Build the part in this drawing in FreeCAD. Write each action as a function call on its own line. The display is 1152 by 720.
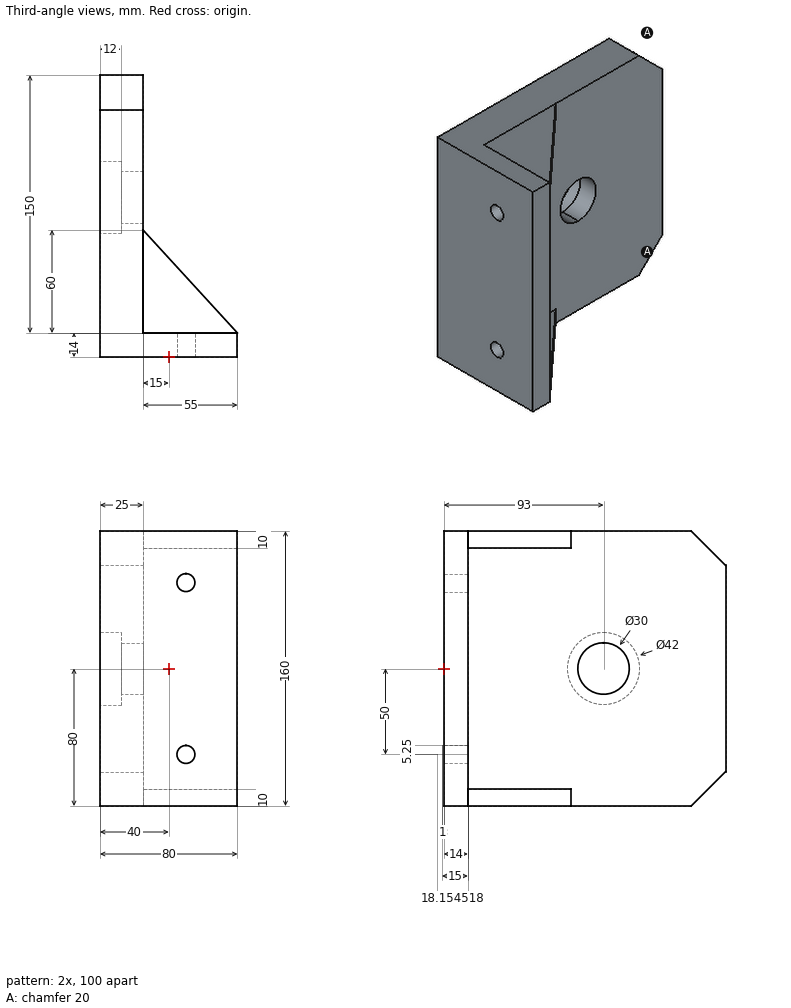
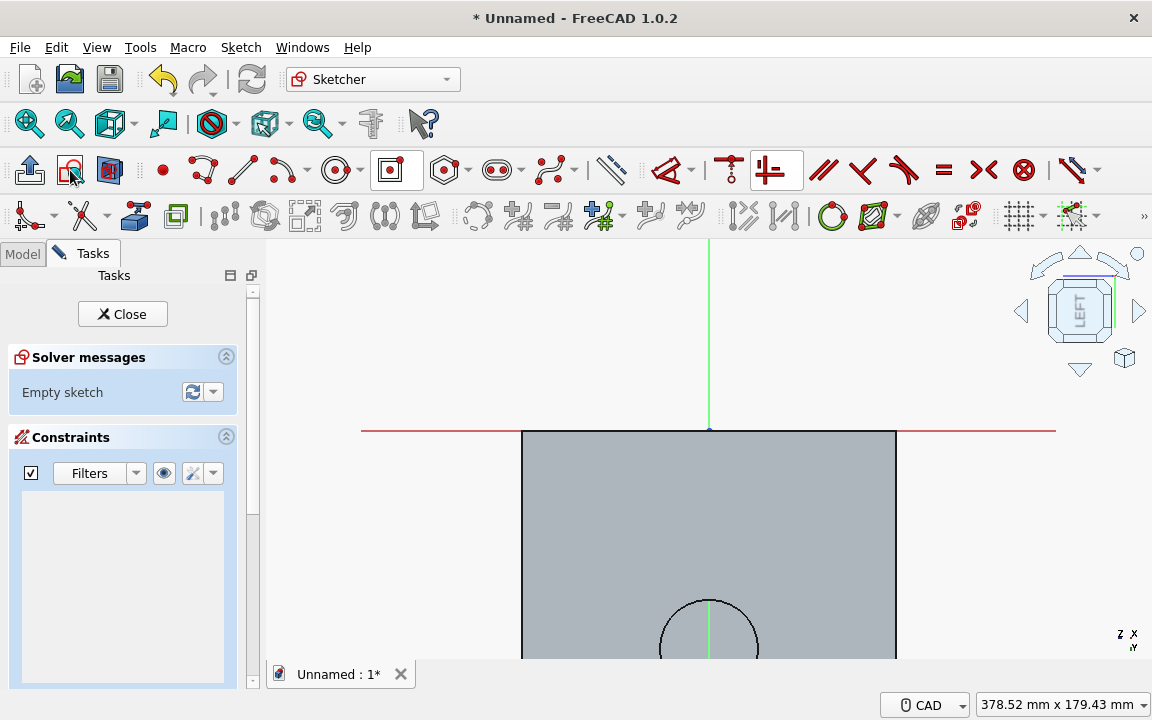
scroll(640, 449, down, 5)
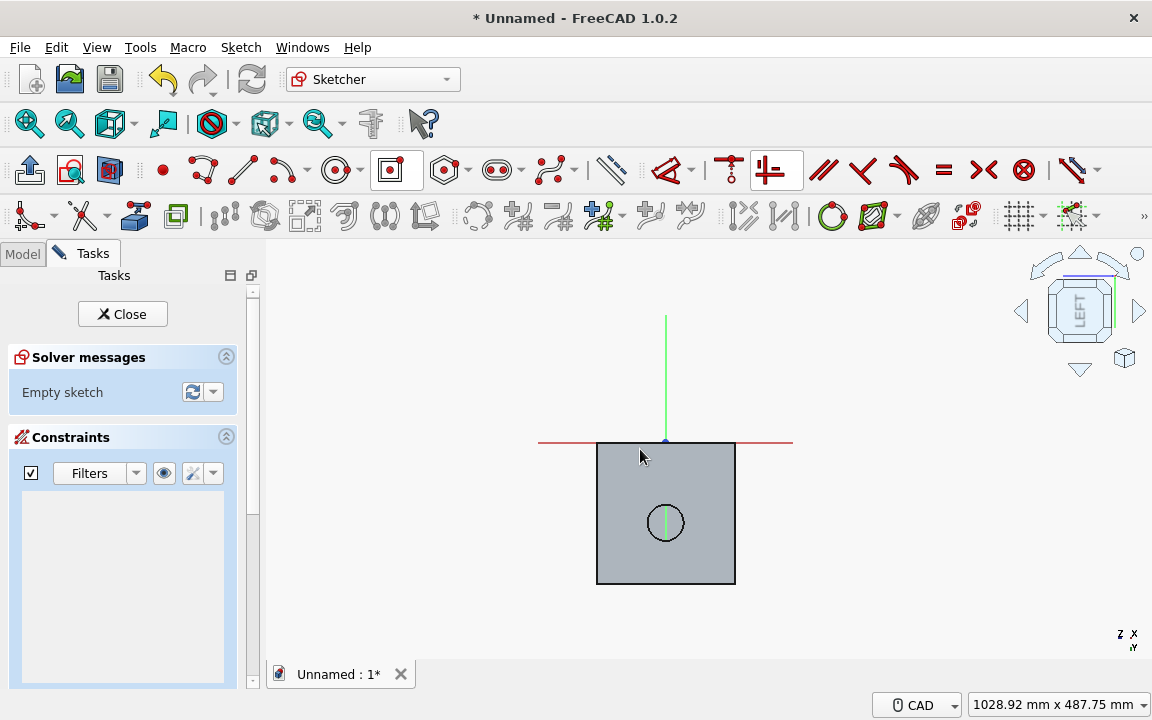
scroll(669, 532, up, 11)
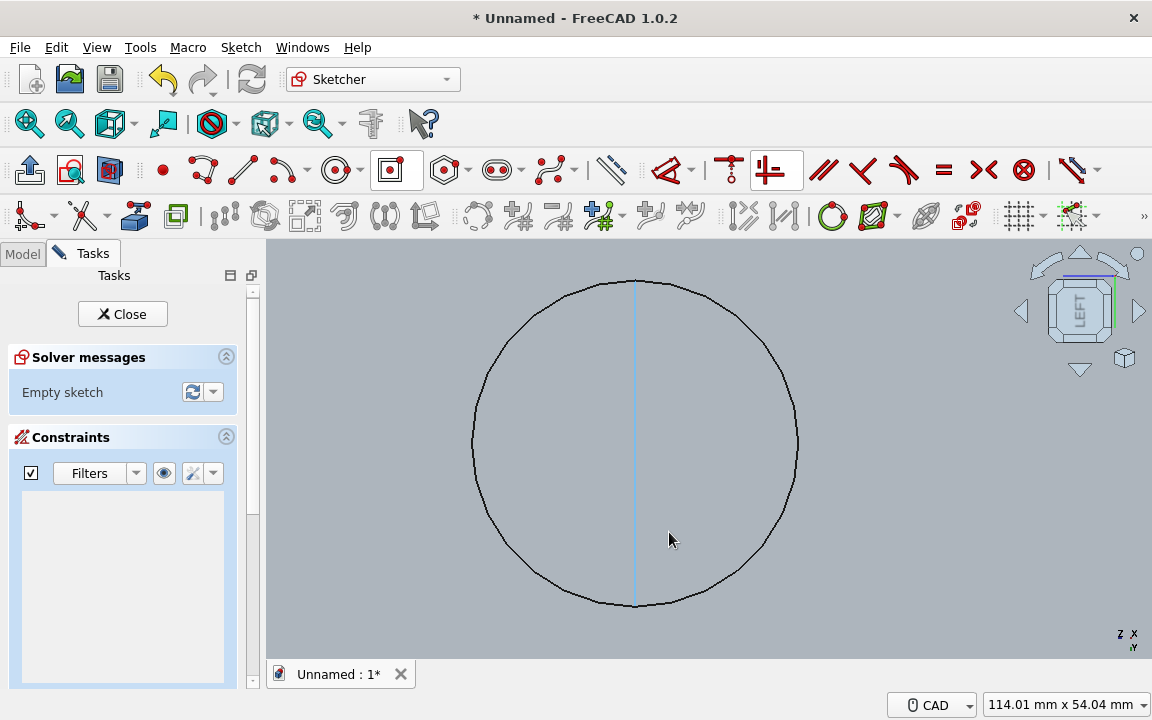
click(336, 170)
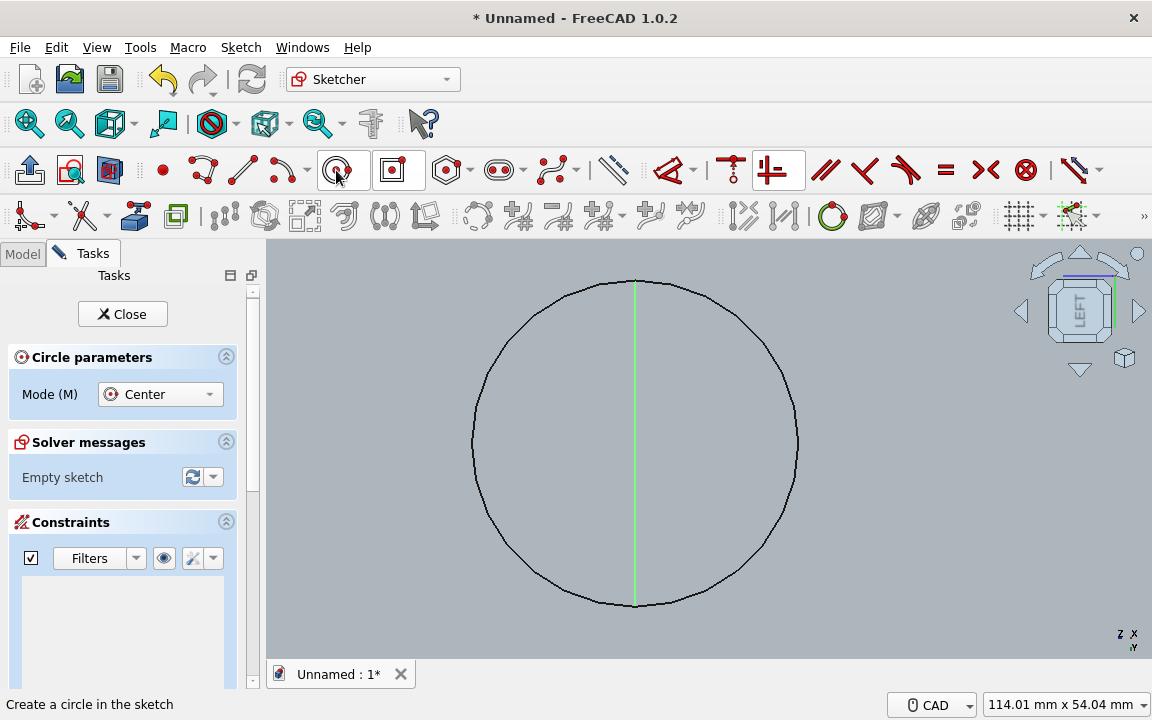
click(635, 444)
move(718, 361)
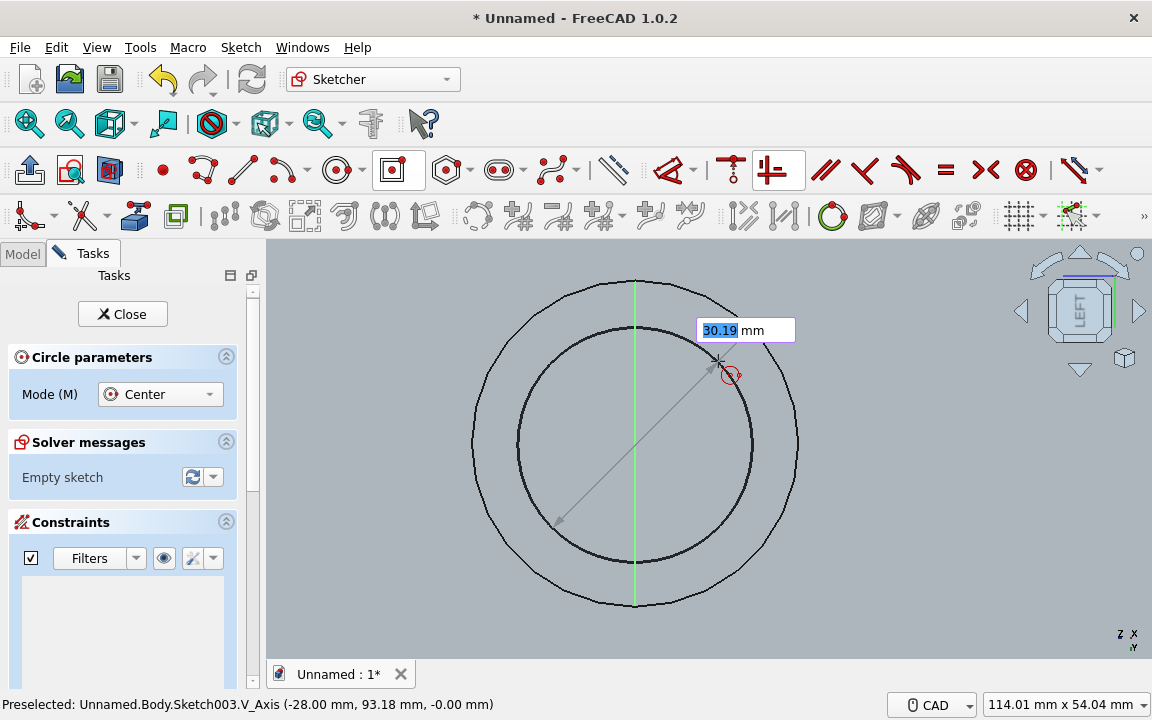
text(30)
key(Return)
key(Escape)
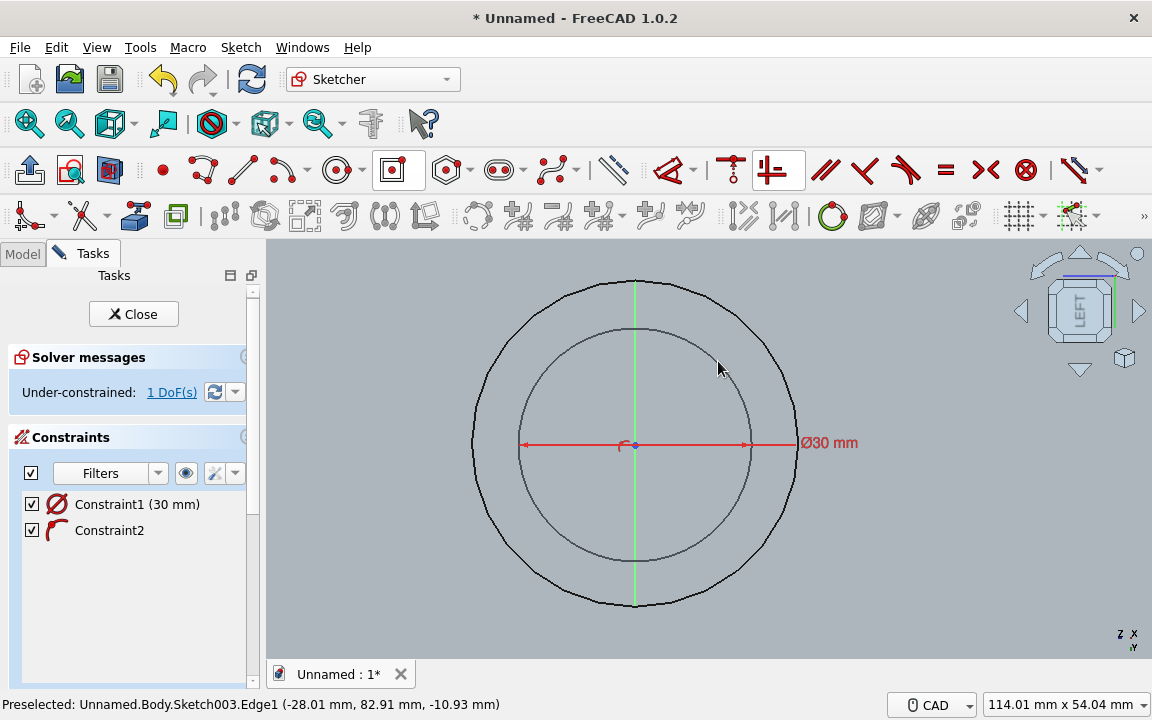
click(668, 170)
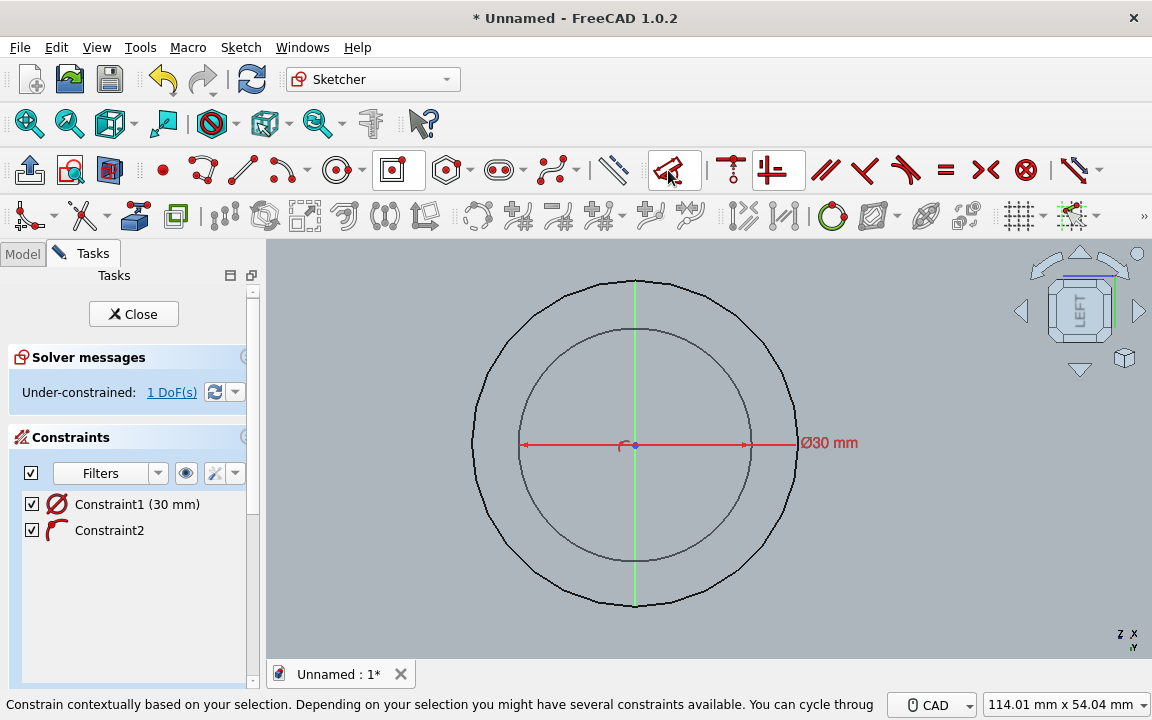
click(635, 445)
click(669, 356)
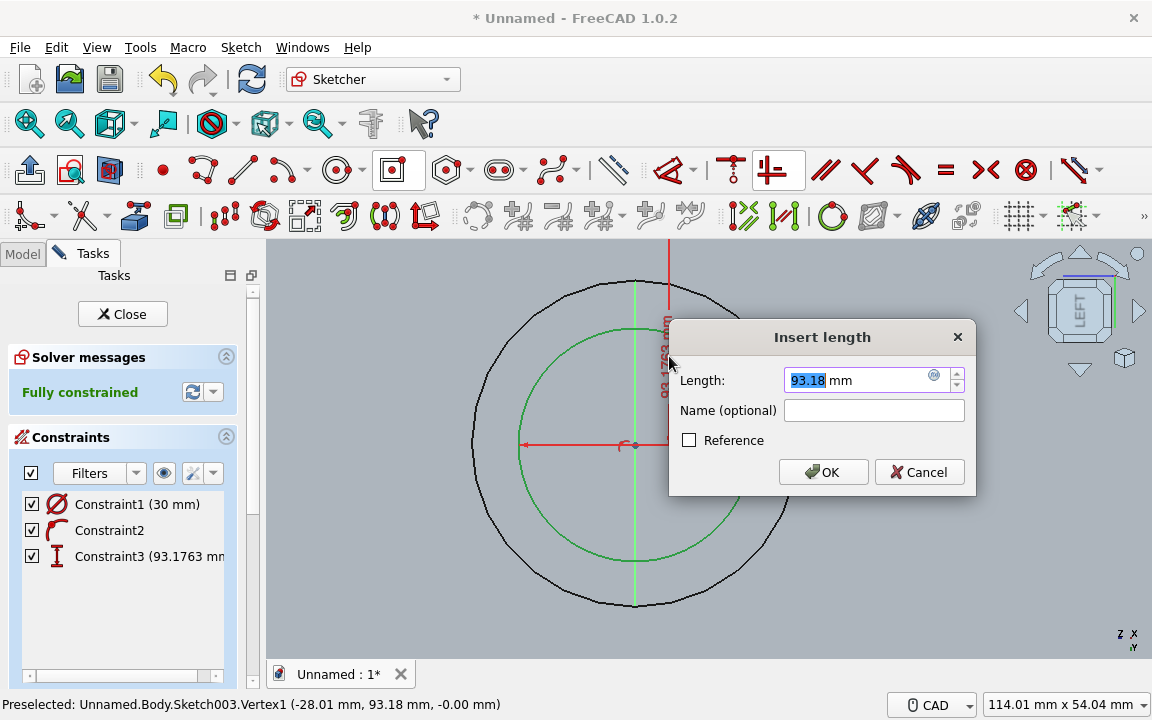
text(93)
key(Return)
key(Escape)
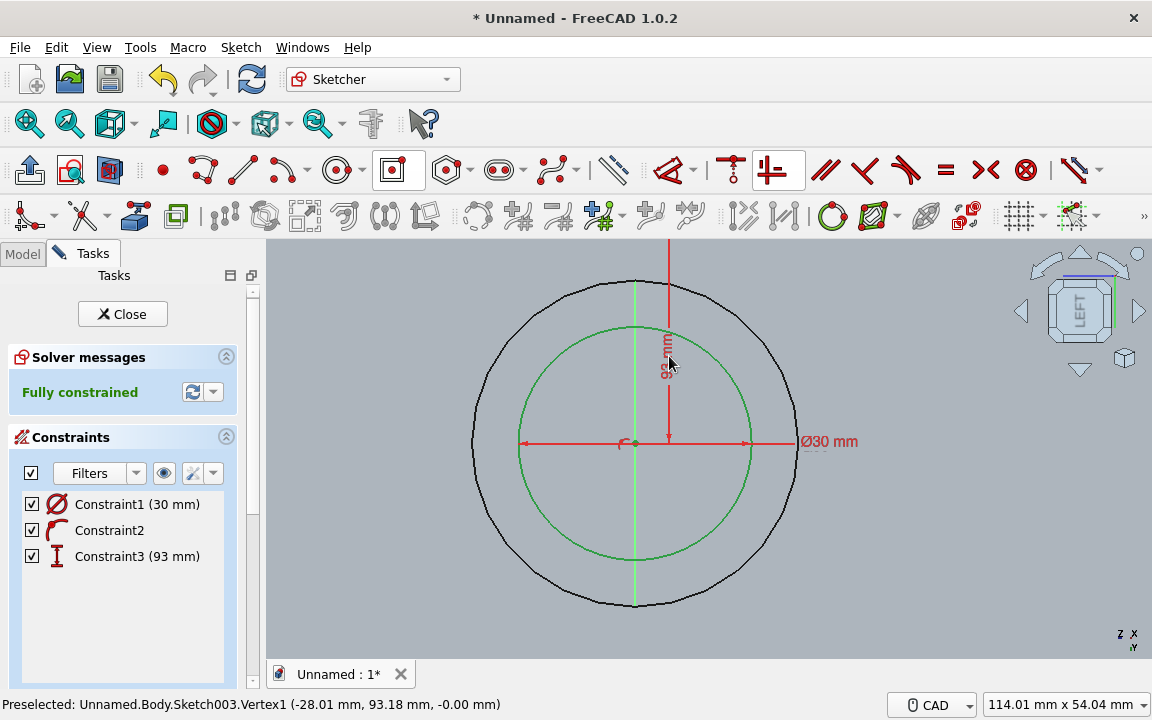
click(123, 314)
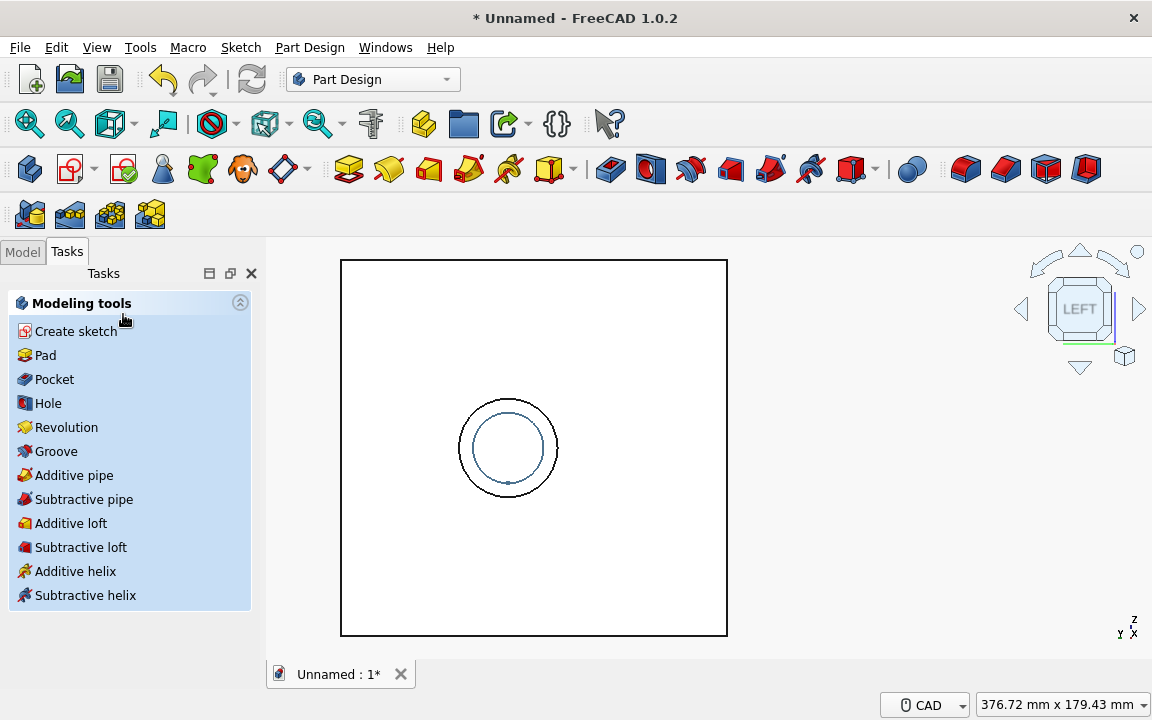
click(612, 170)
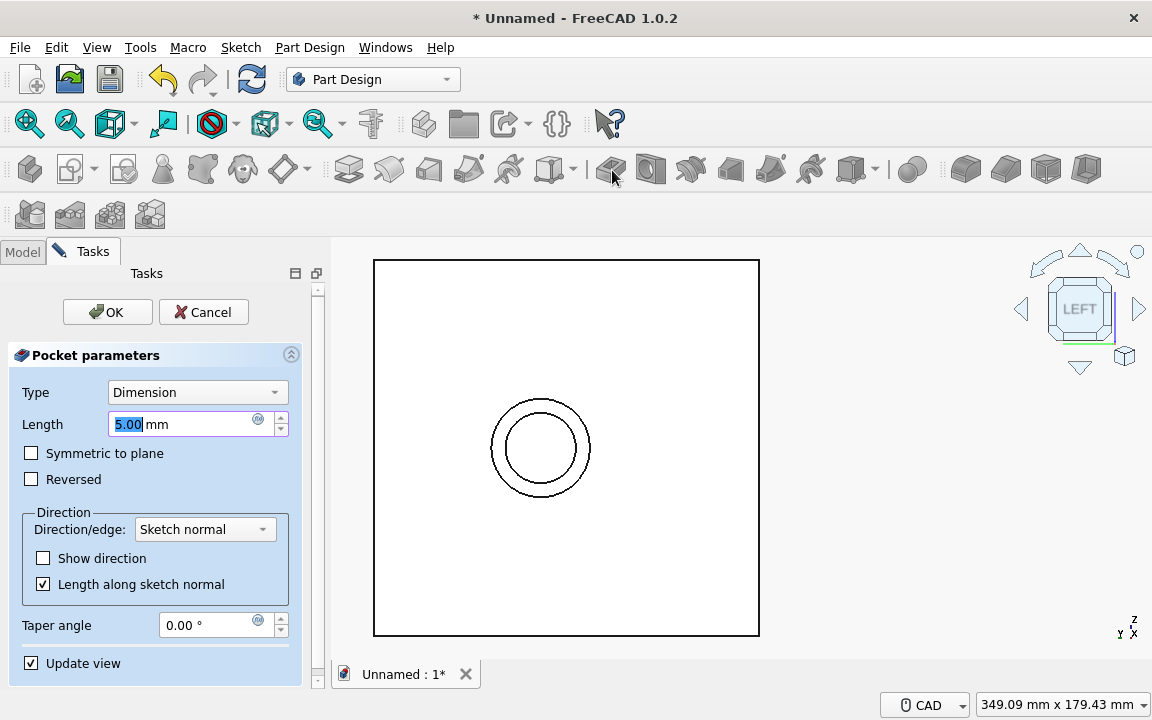
click(198, 392)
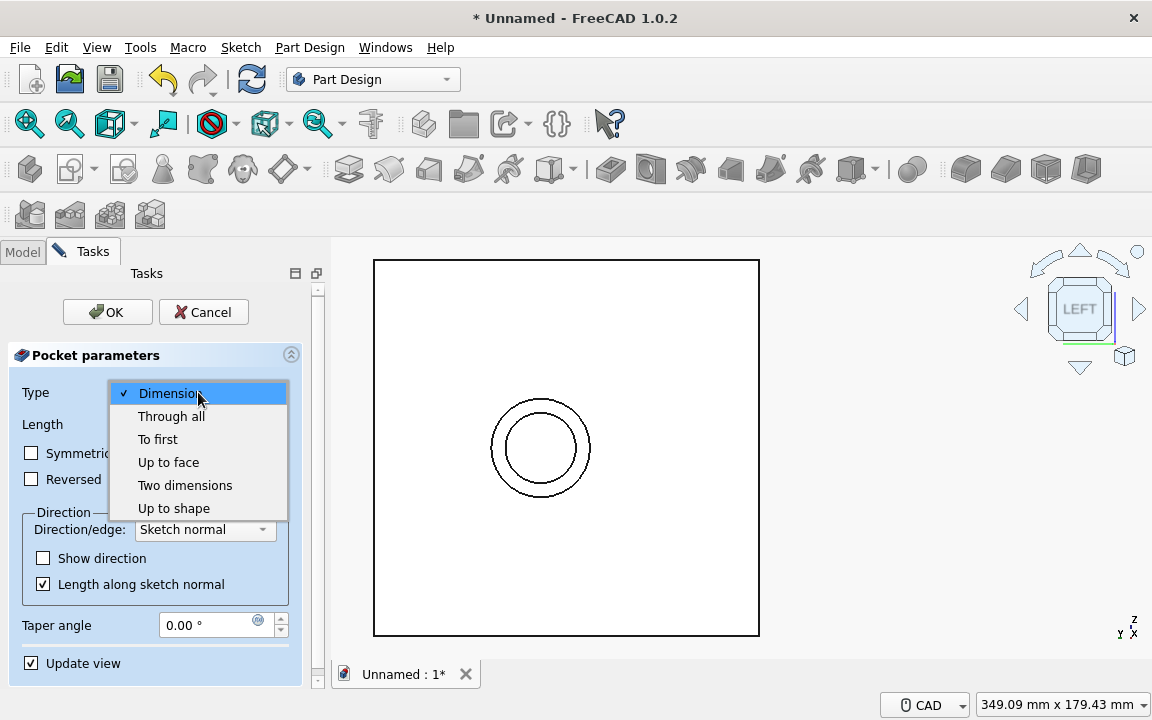
click(198, 416)